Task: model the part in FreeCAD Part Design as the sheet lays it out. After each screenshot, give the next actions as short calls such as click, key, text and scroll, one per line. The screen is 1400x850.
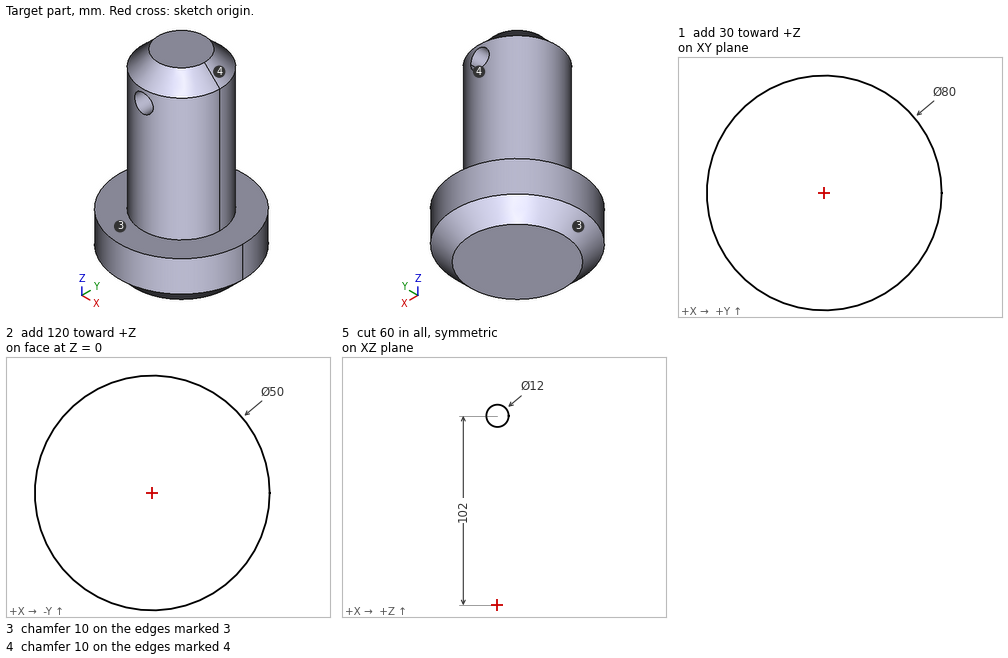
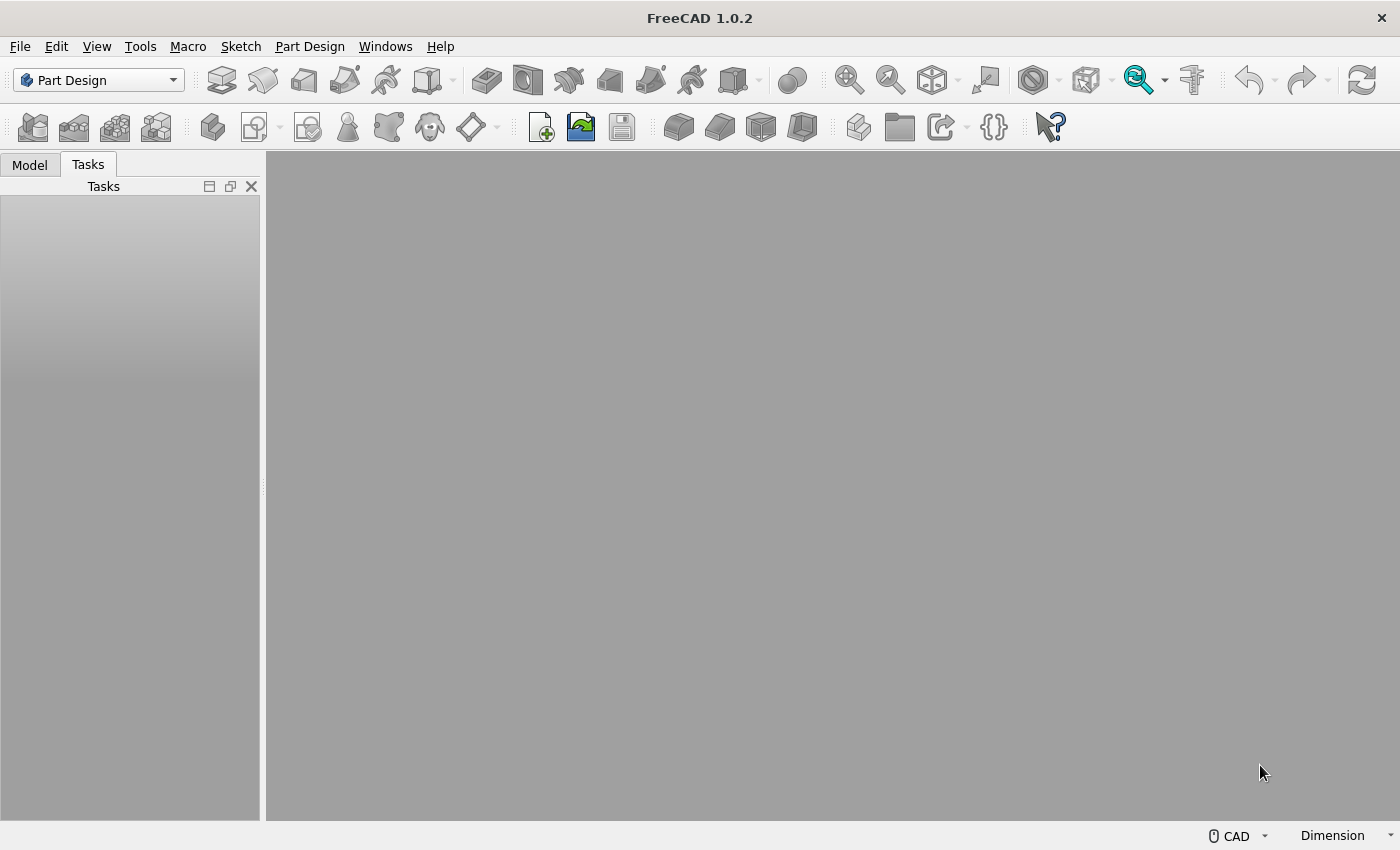
click(540, 128)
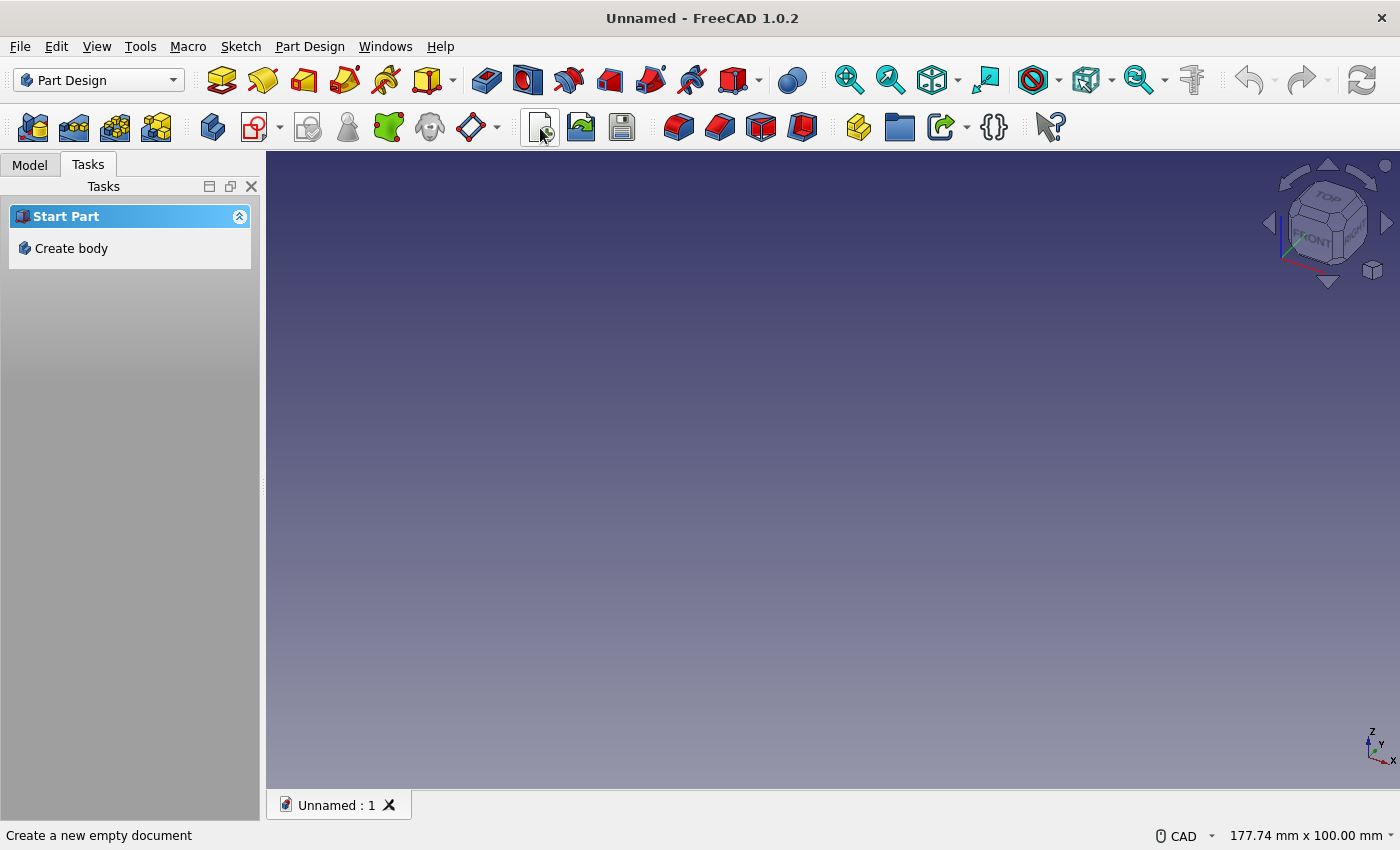
click(254, 128)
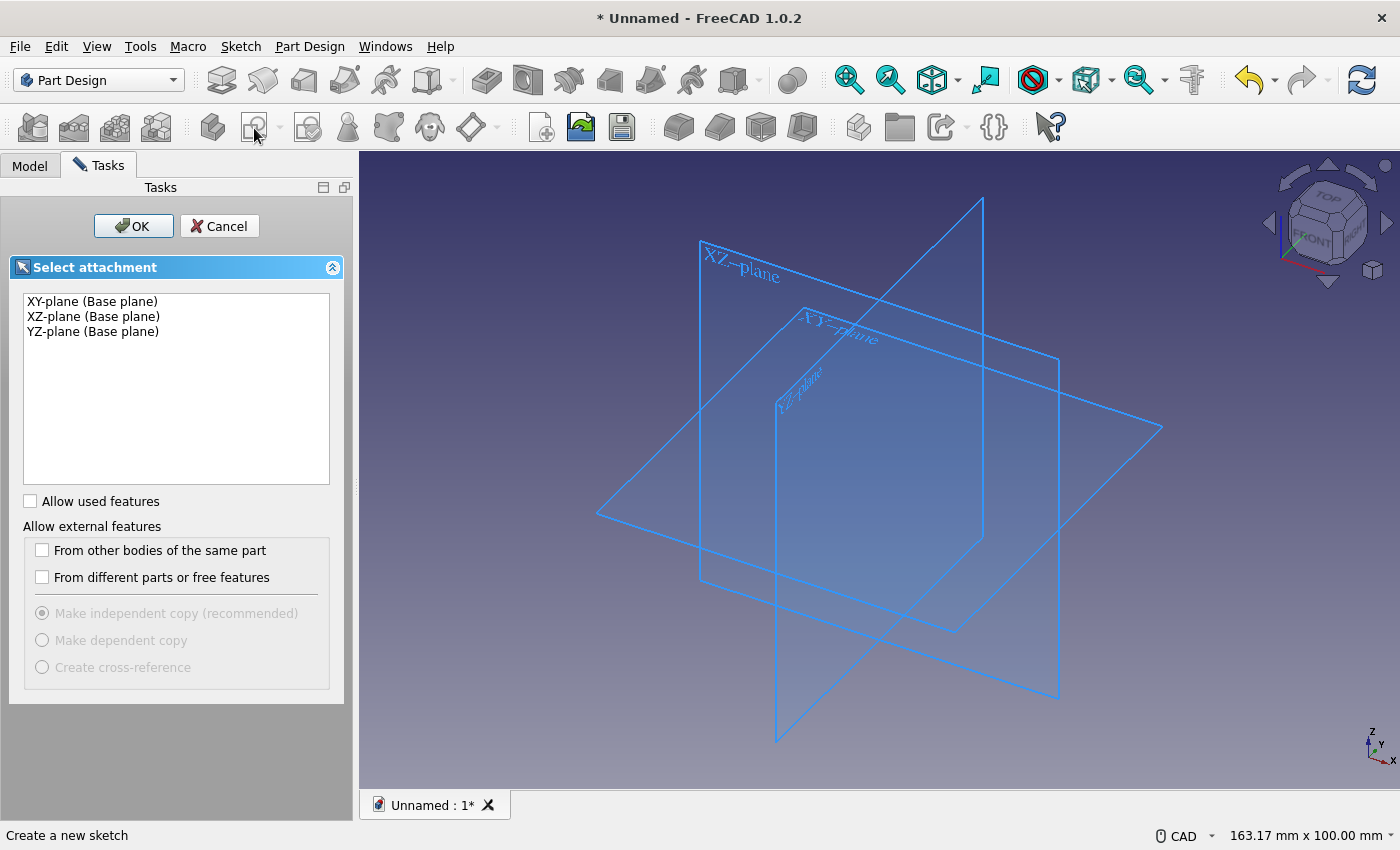
click(84, 302)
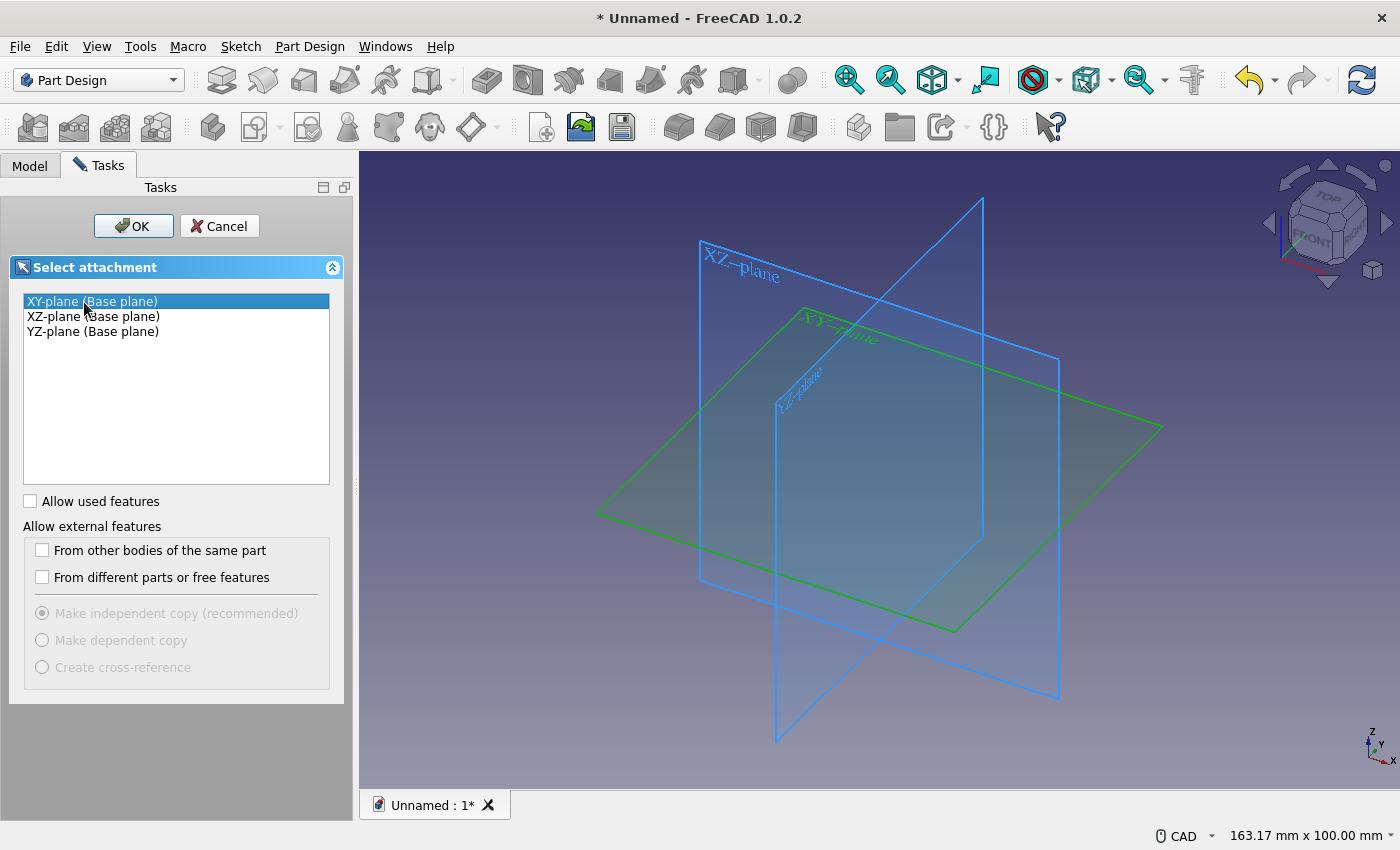
click(134, 226)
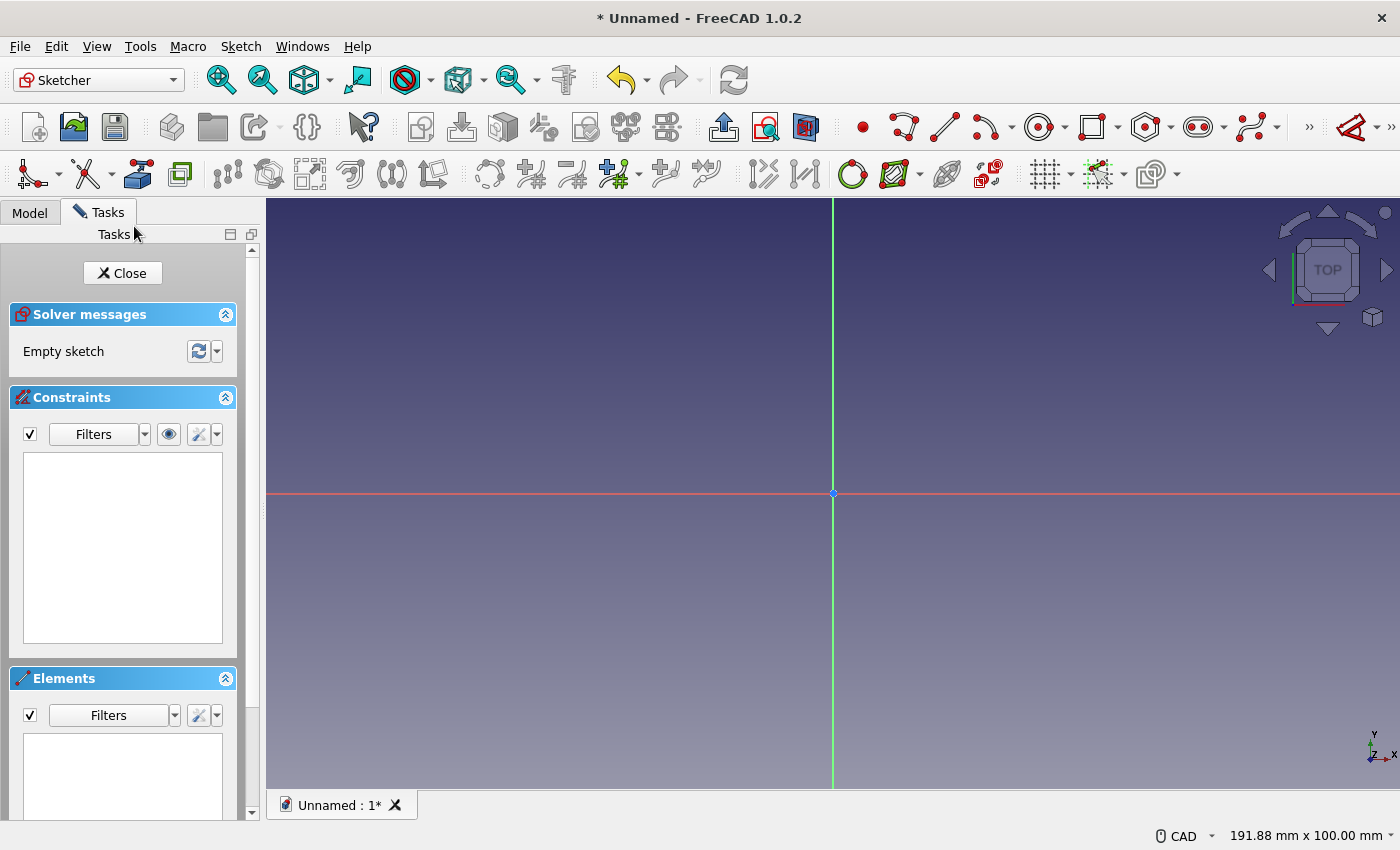
key(g)
key(c)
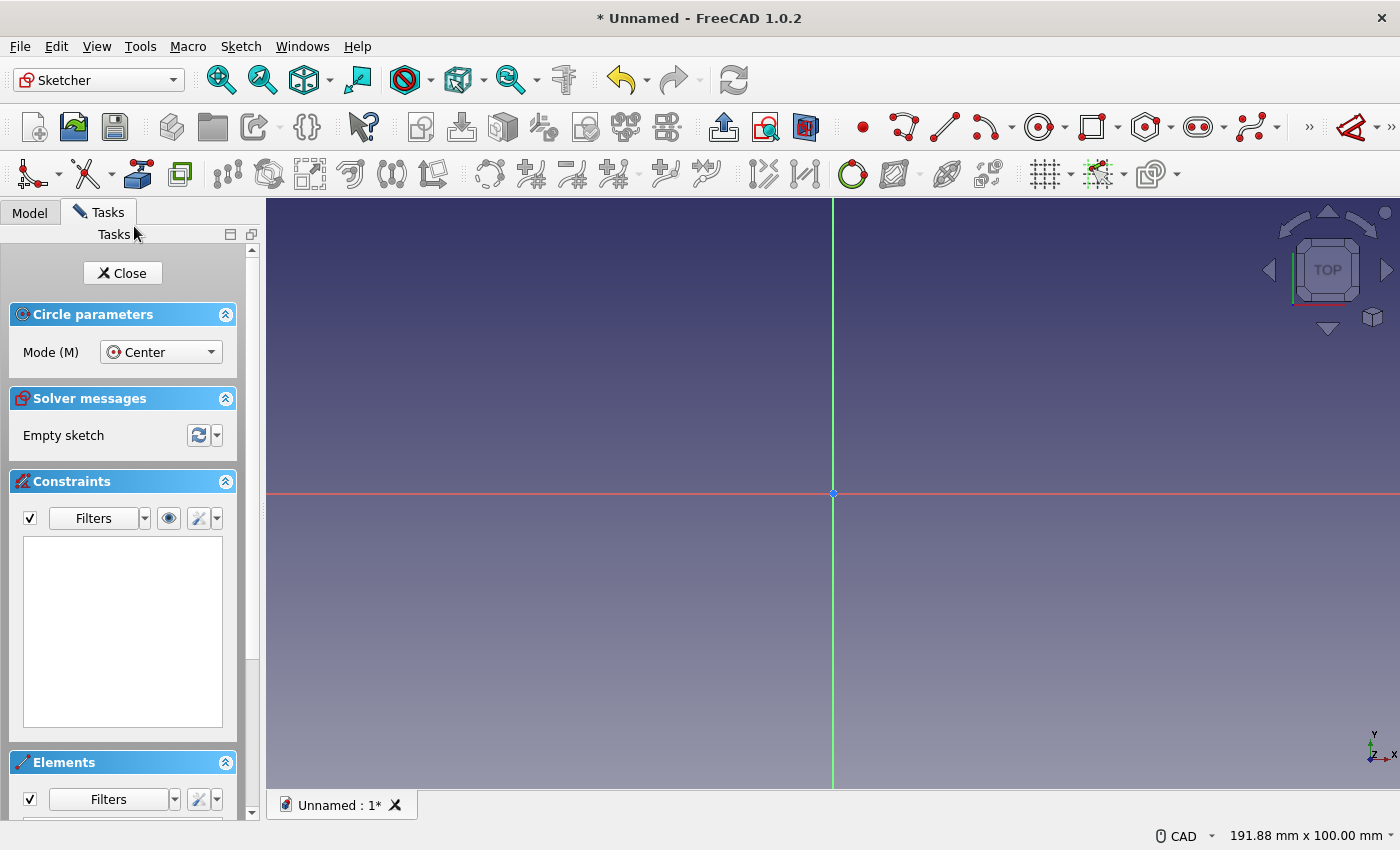
click(833, 494)
click(1000, 326)
key(Escape)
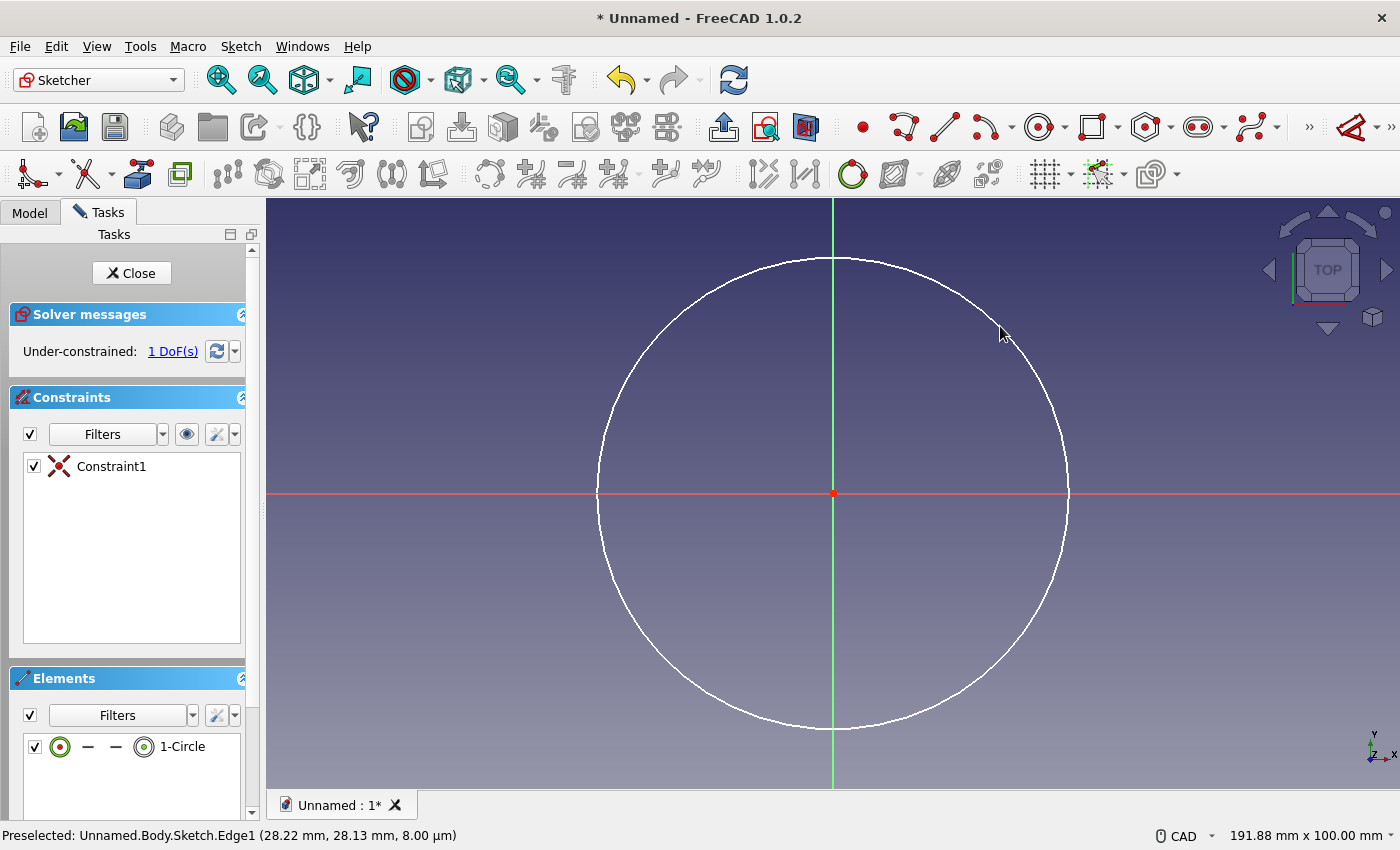
key(d)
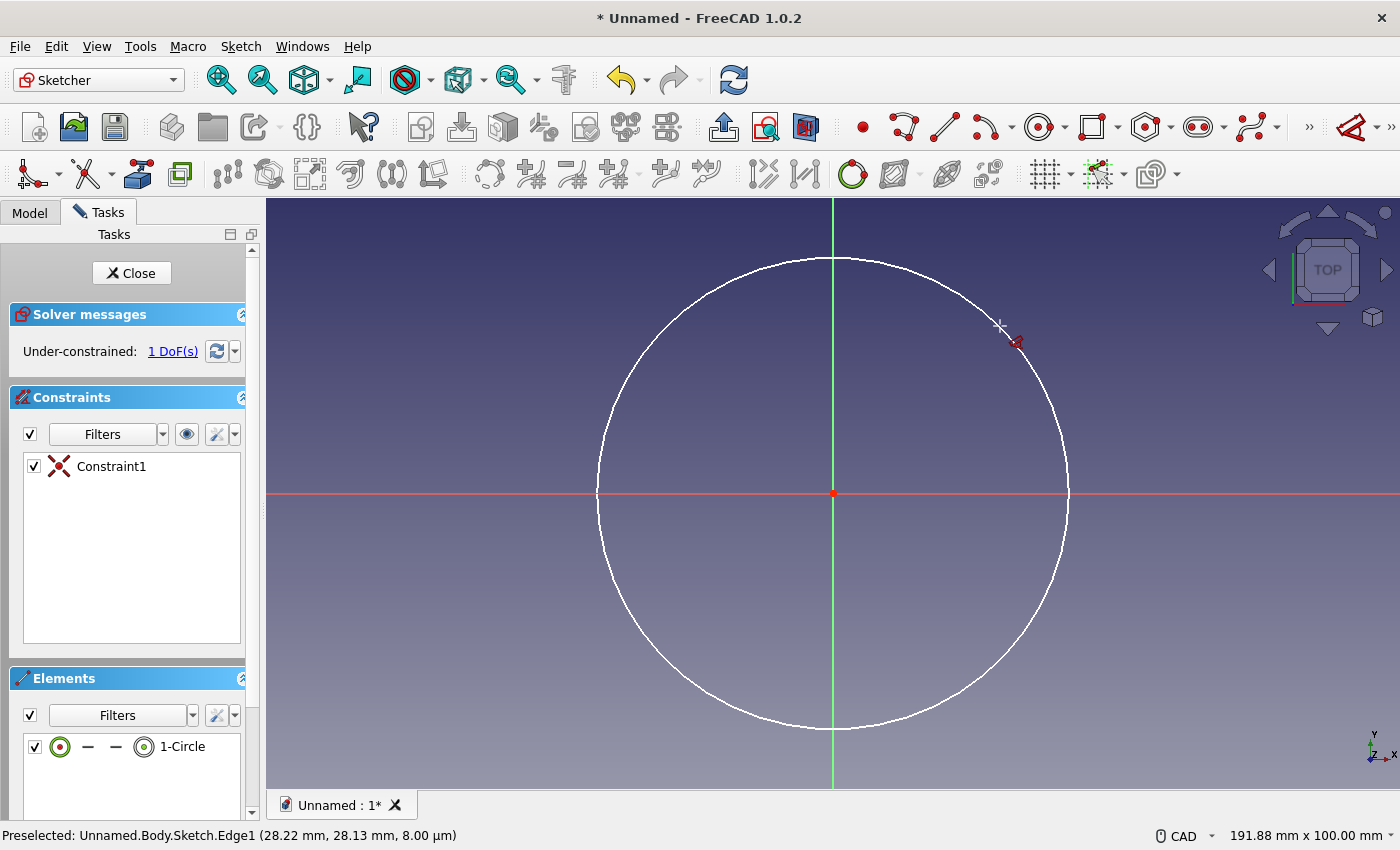
click(999, 326)
click(1022, 303)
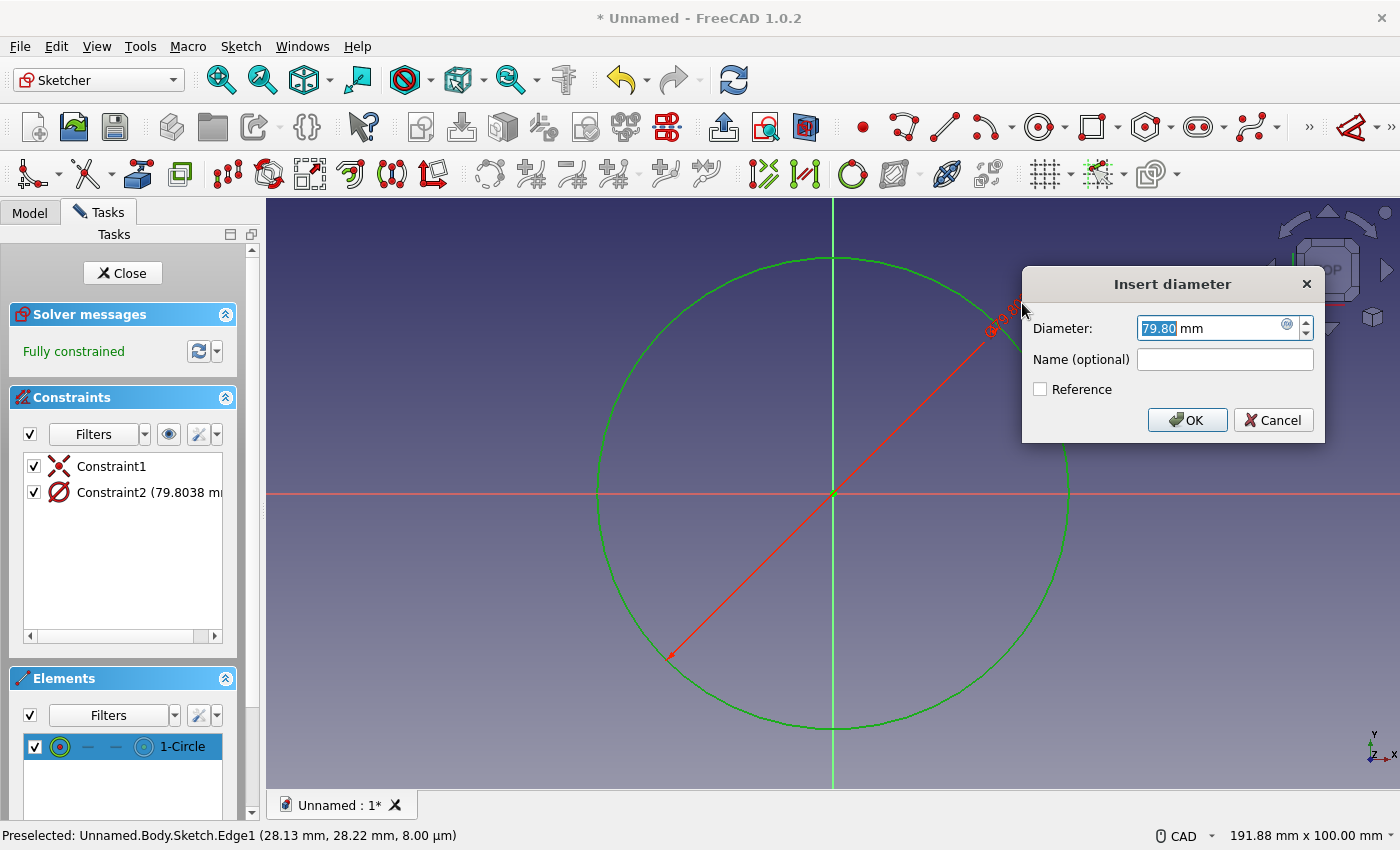
text(80)
key(Return)
key(Escape)